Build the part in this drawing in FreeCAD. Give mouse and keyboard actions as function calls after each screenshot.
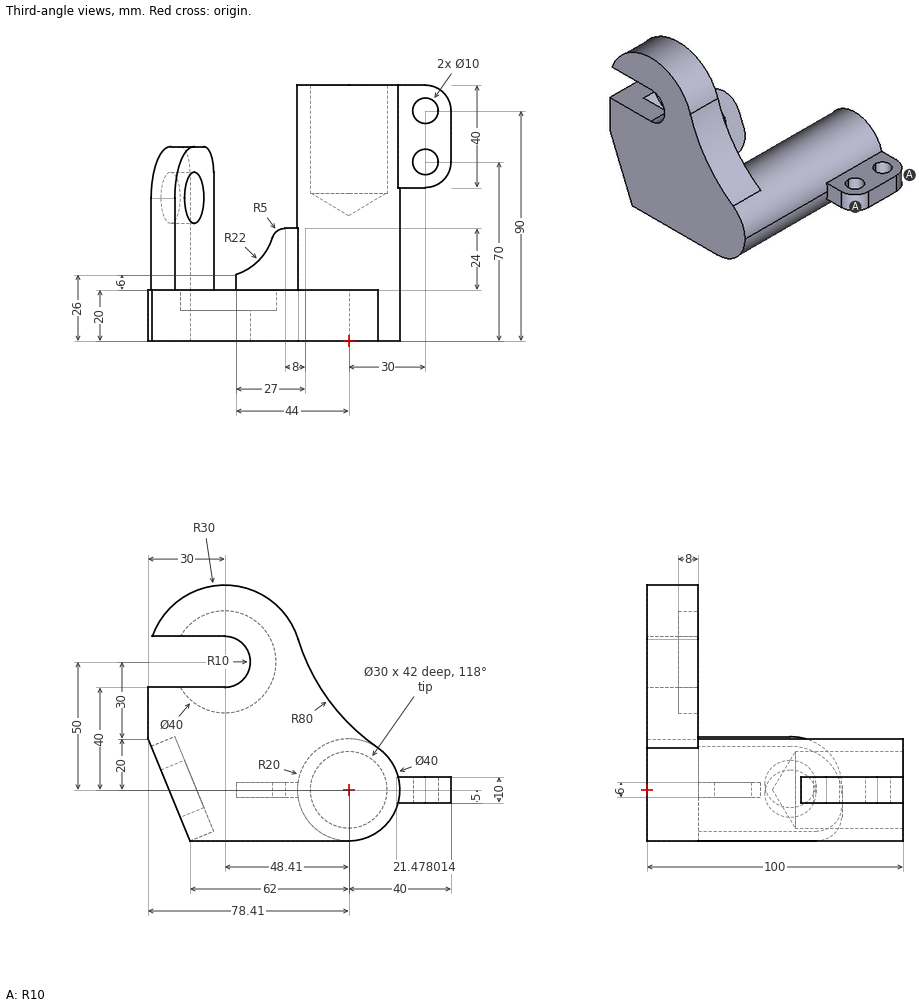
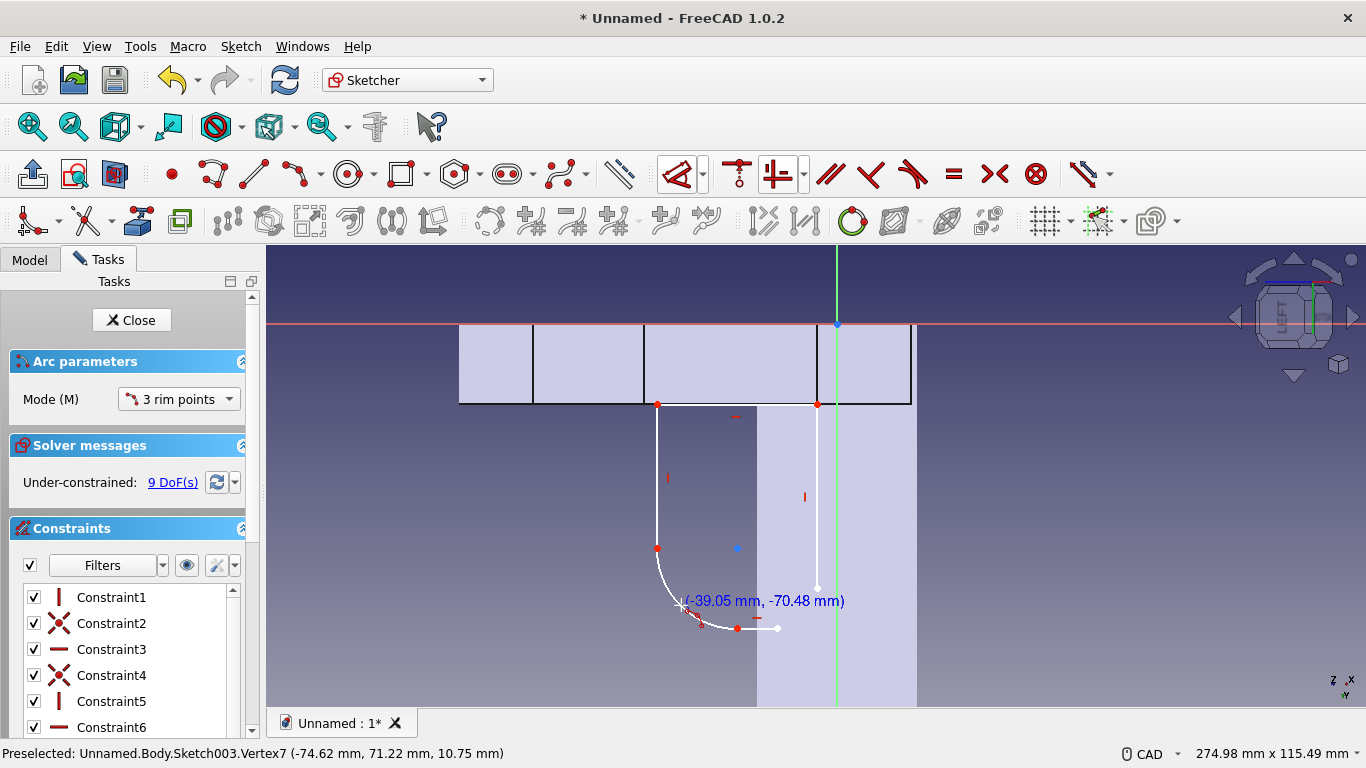
click(777, 629)
click(817, 589)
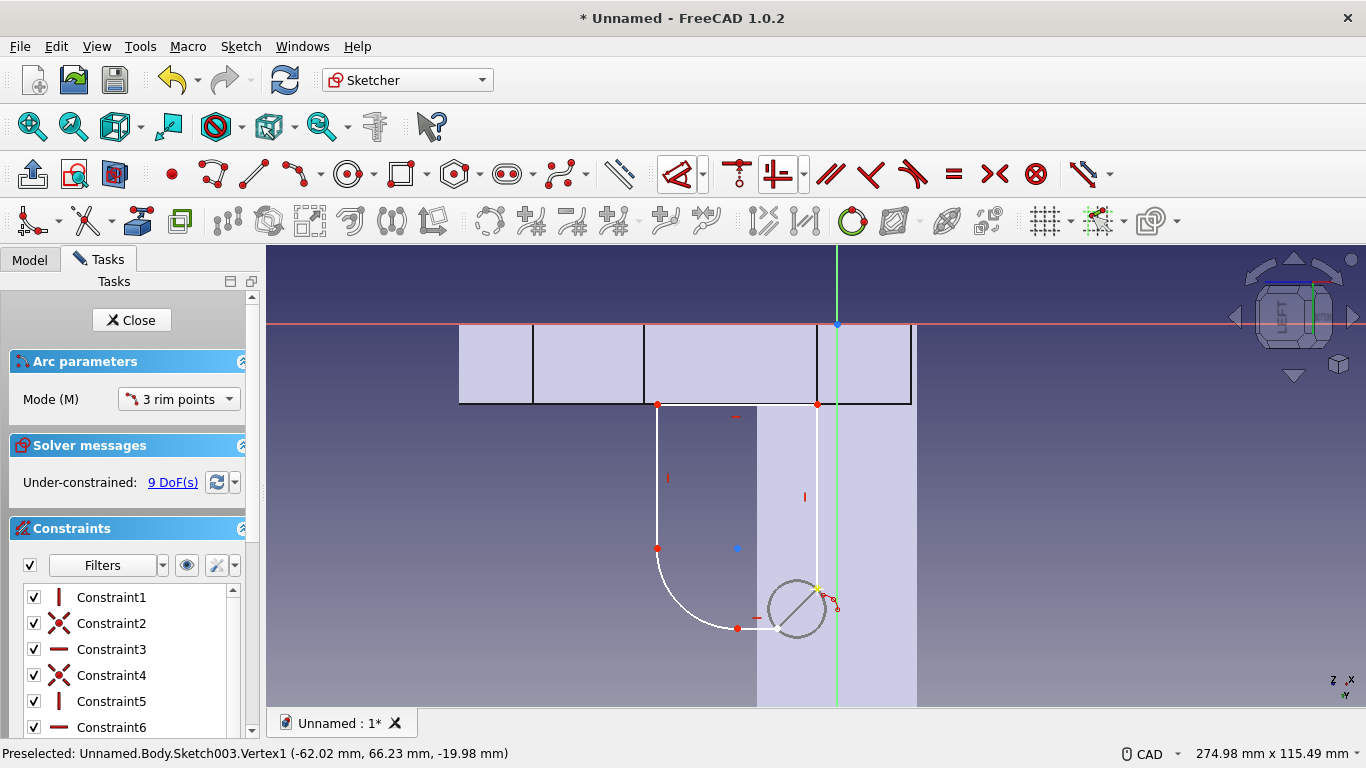
scroll(805, 616, up, 2)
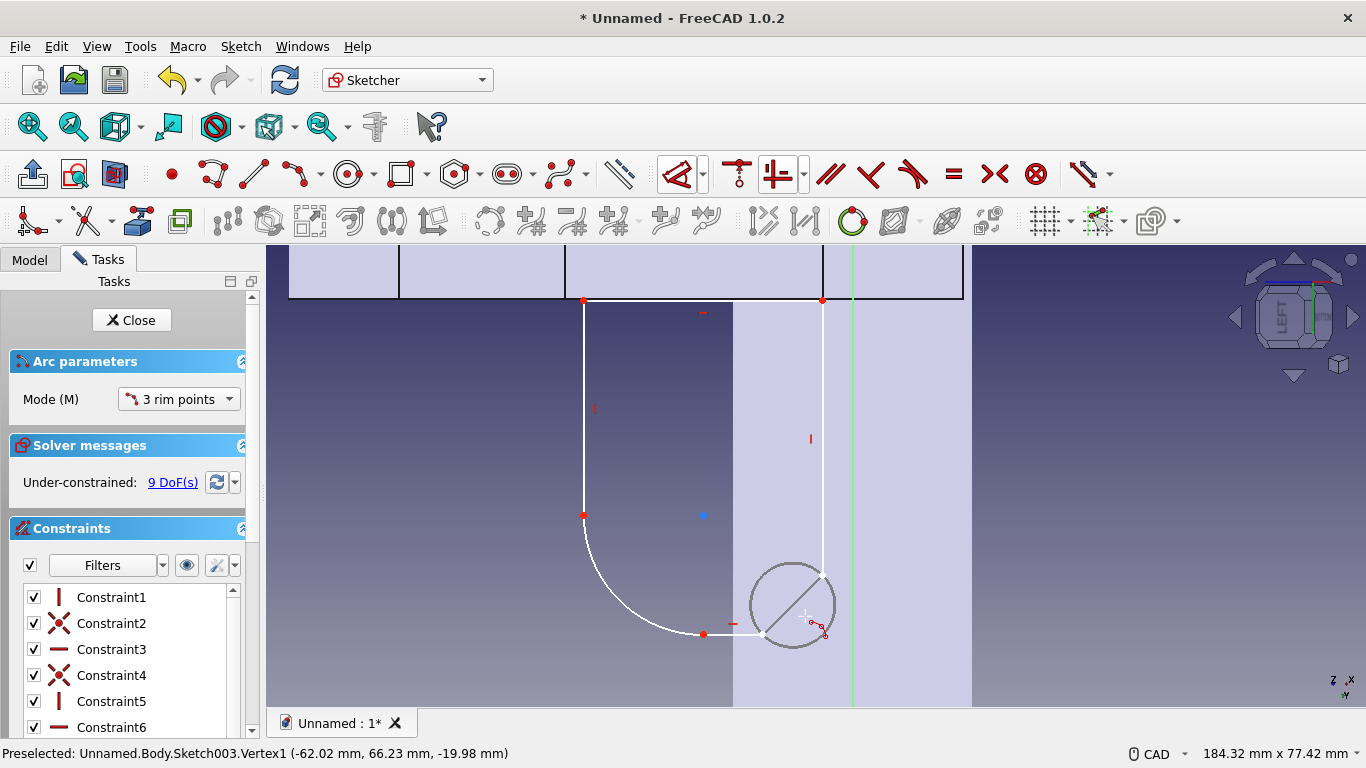
click(805, 616)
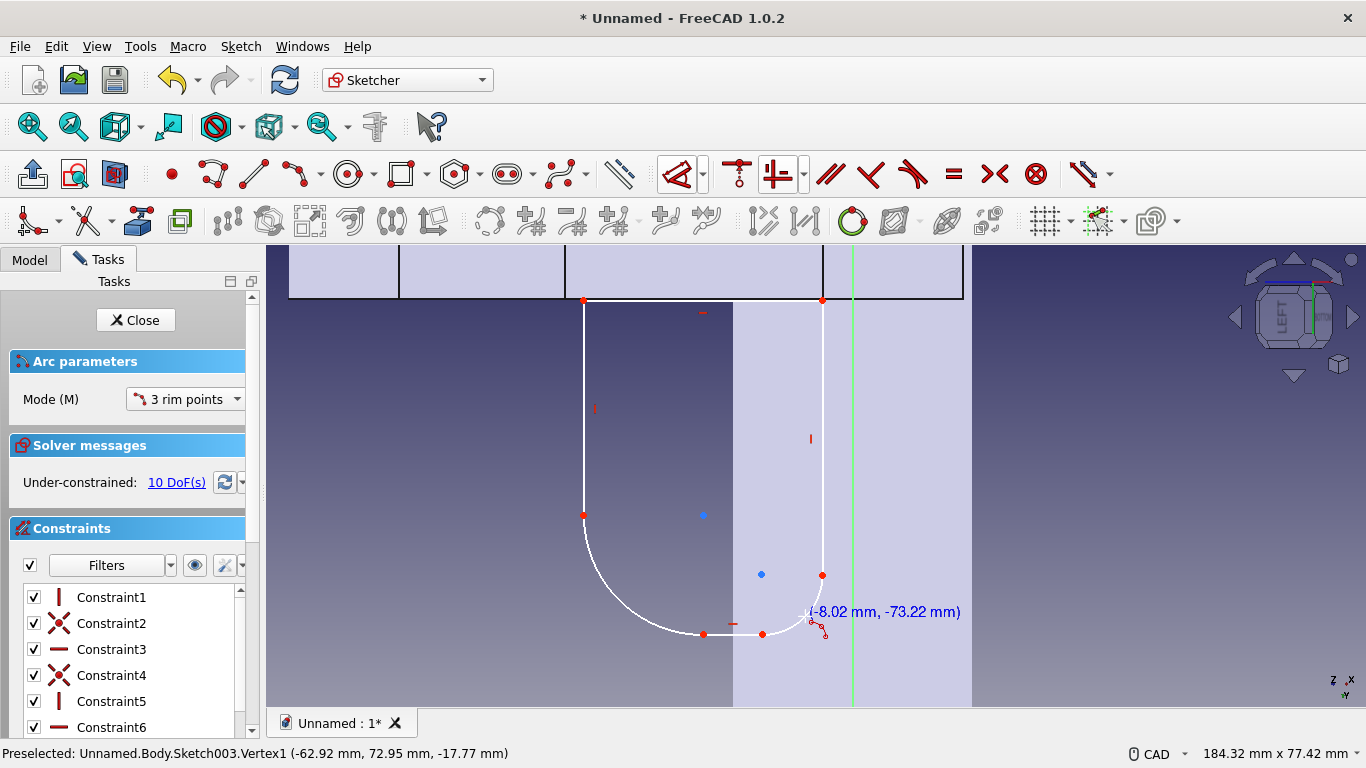
key(g)
key(c)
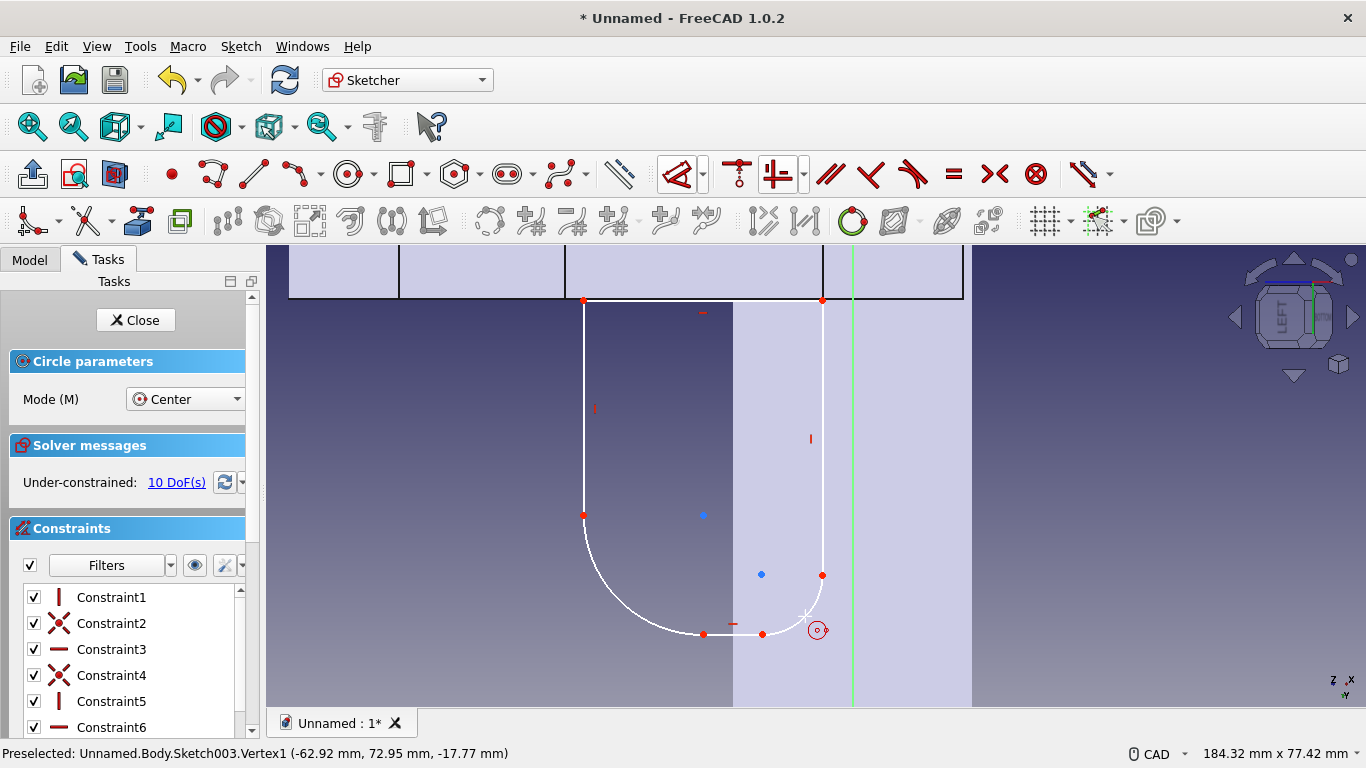
click(703, 514)
click(746, 472)
key(Escape)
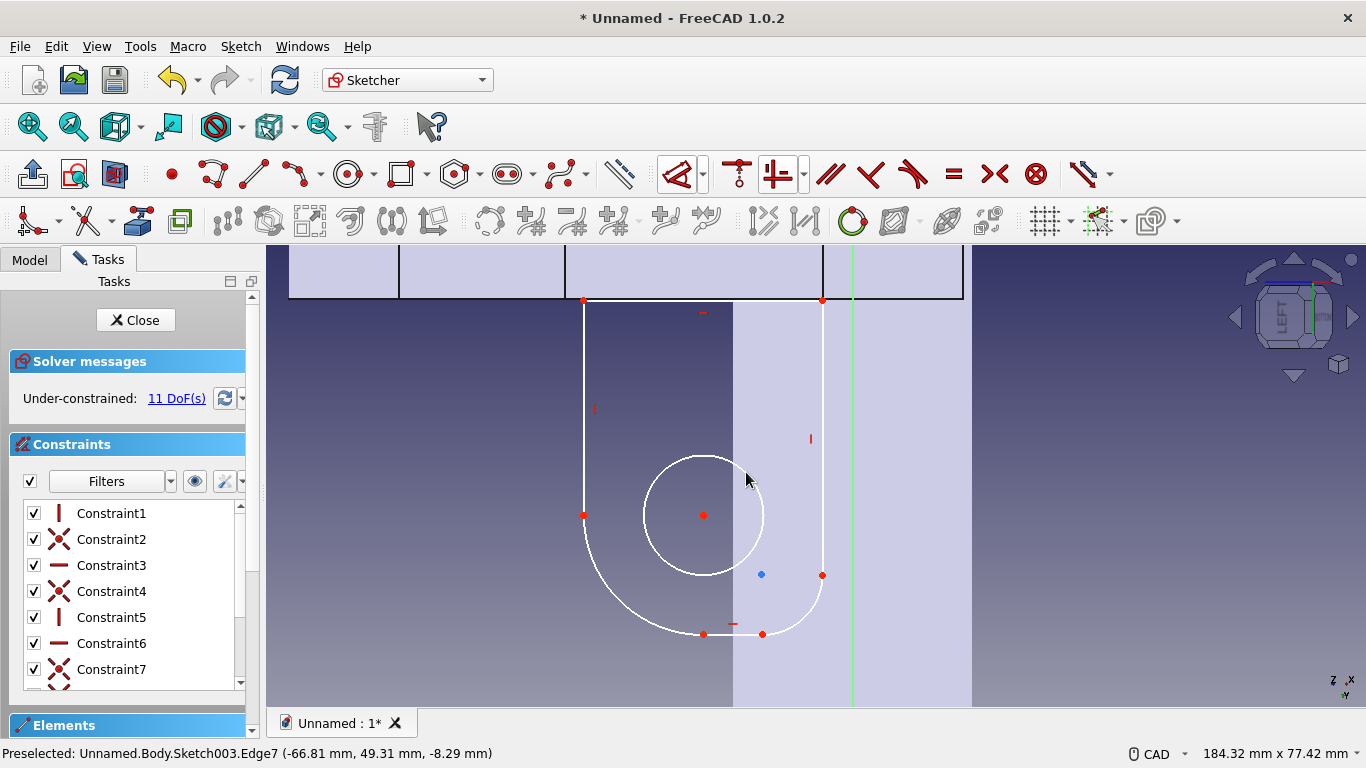
click(823, 493)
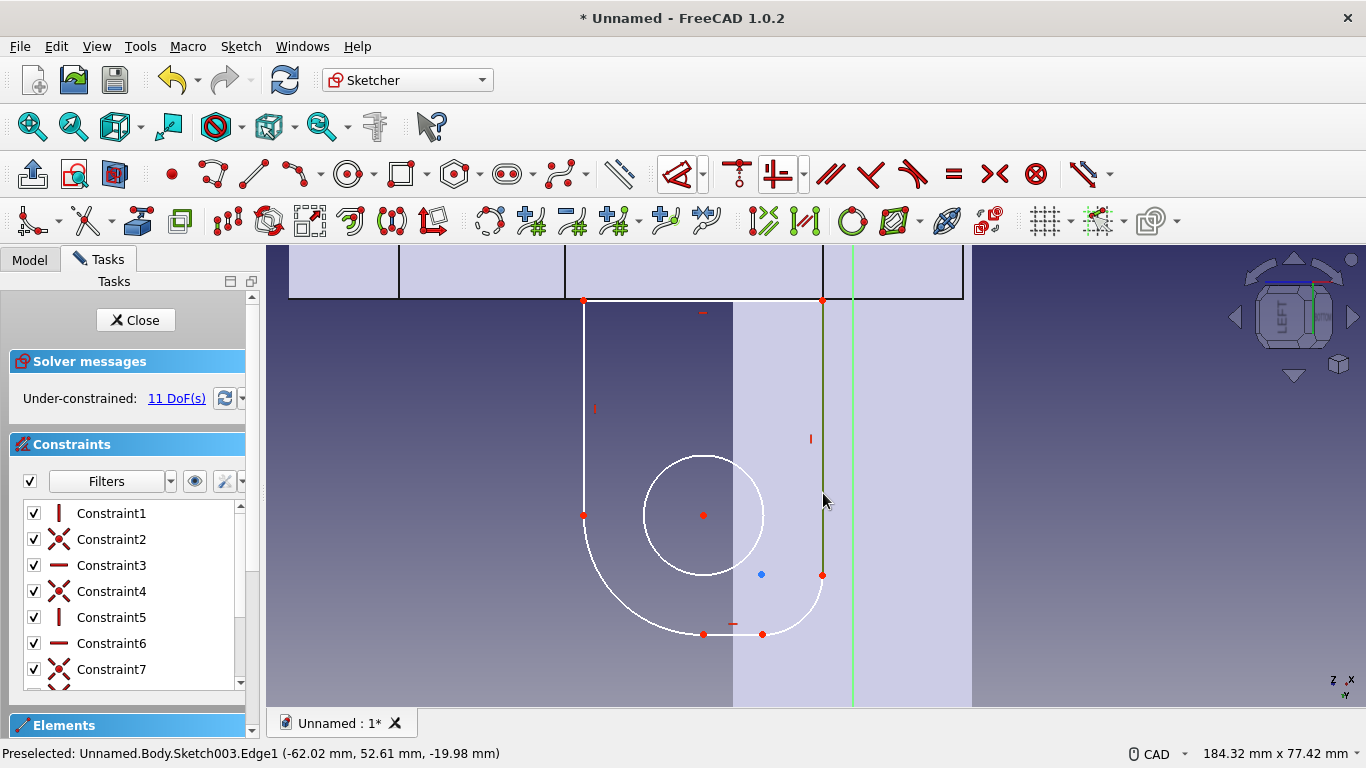
click(790, 628)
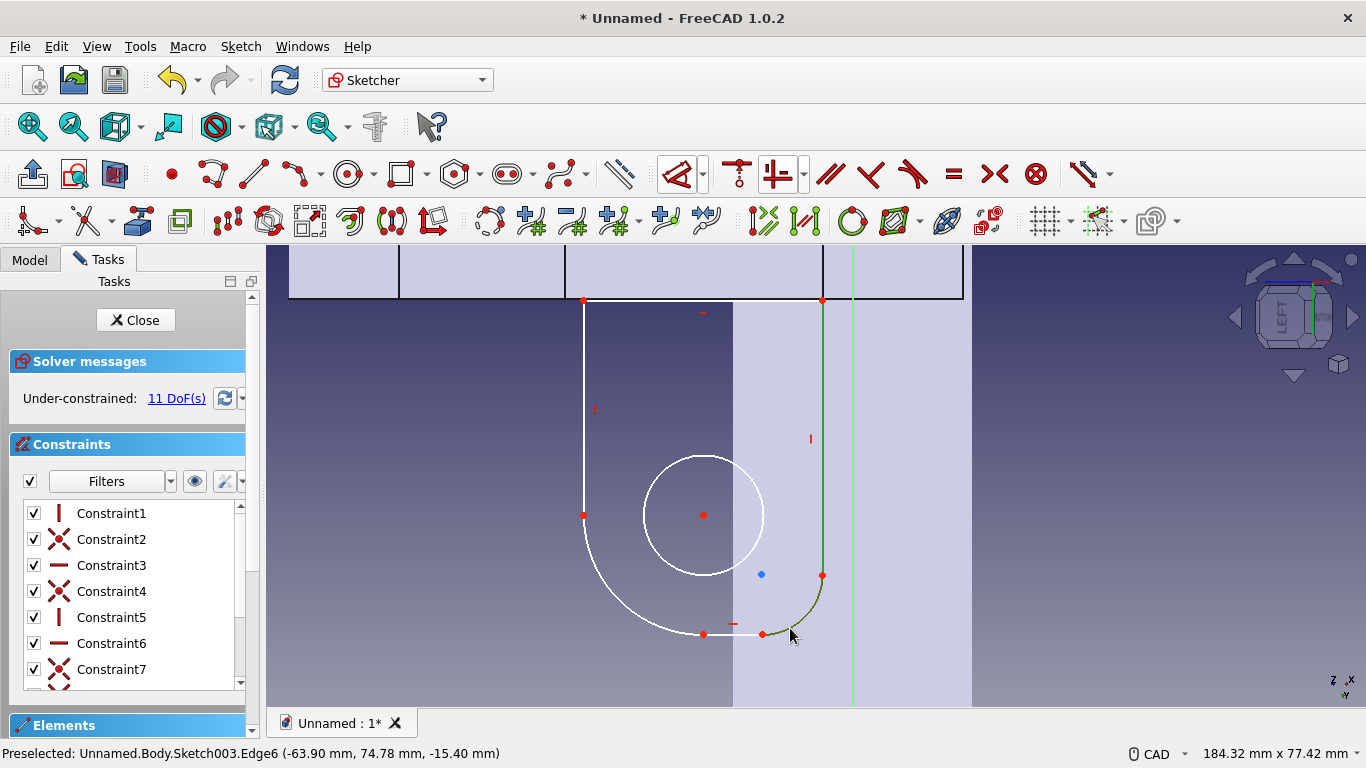
key(t)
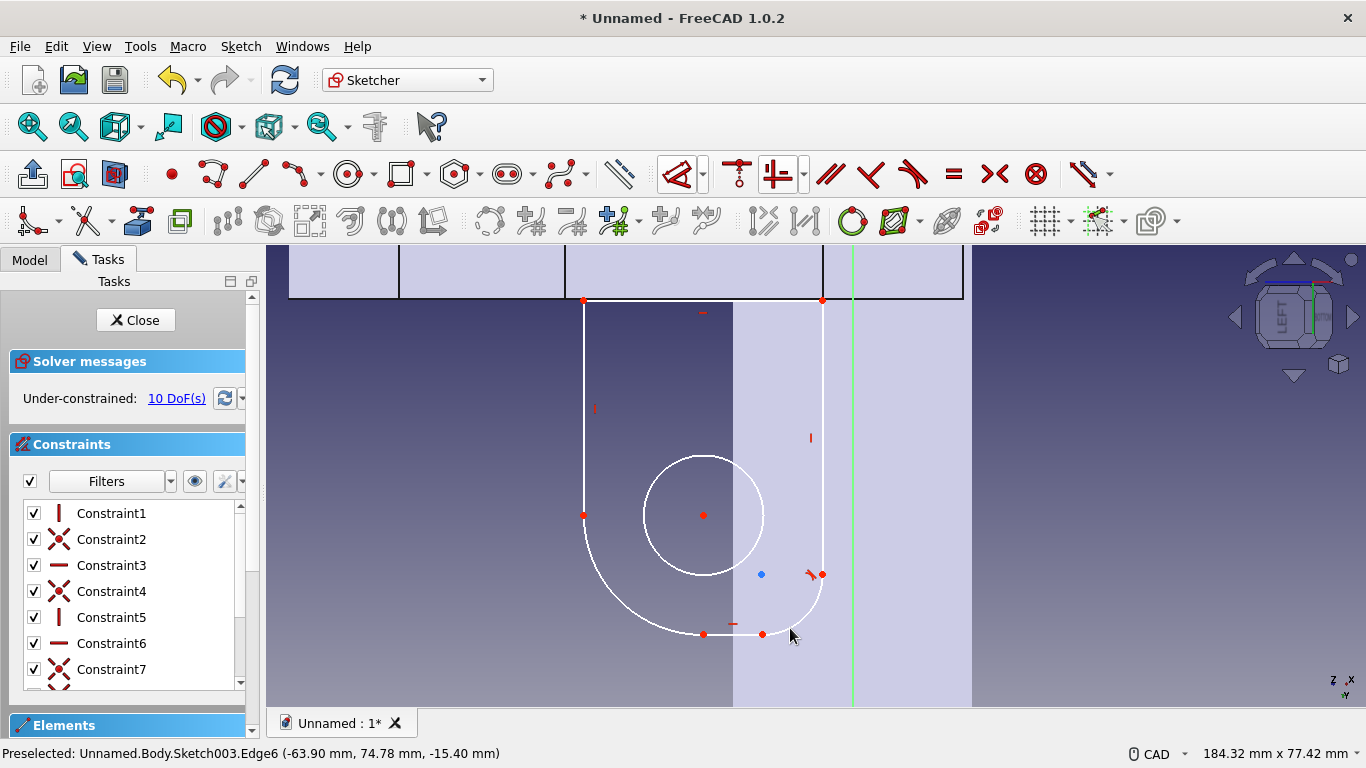
click(584, 365)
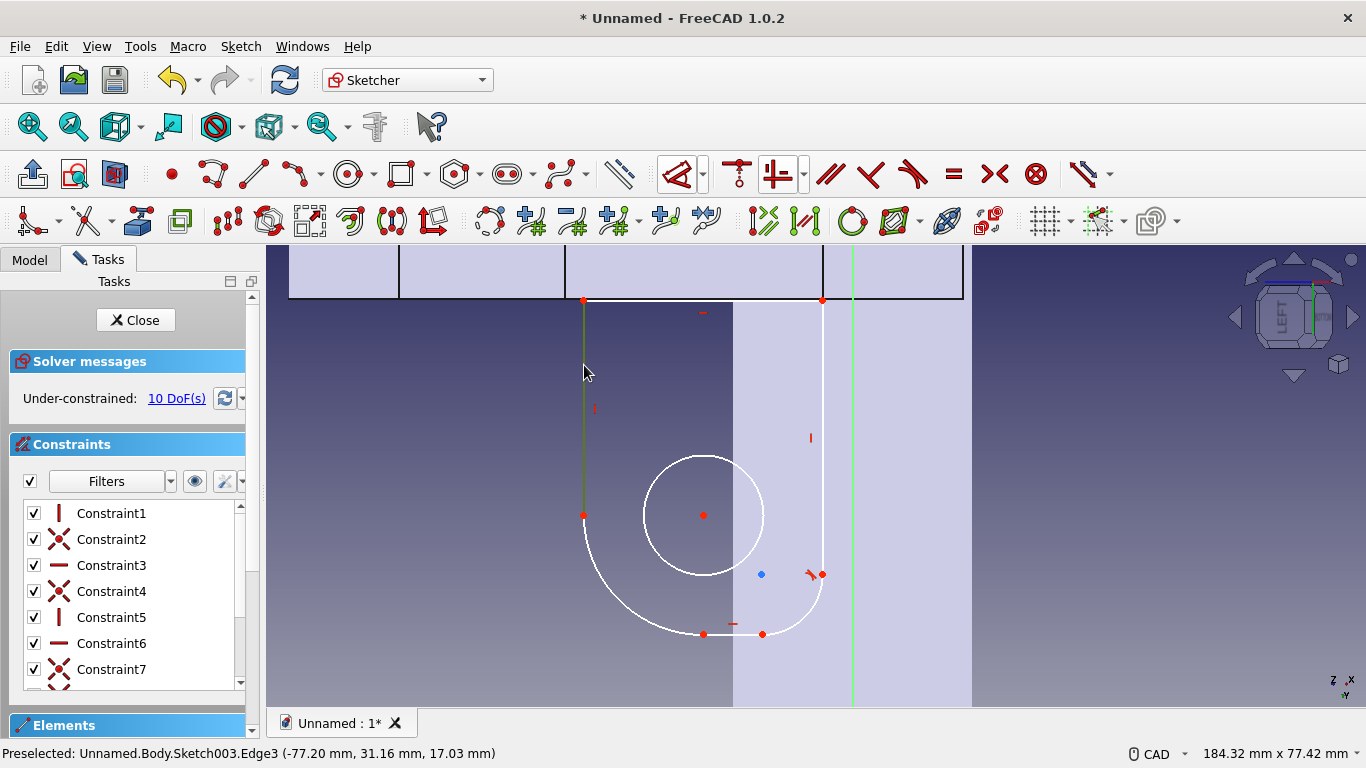
click(597, 570)